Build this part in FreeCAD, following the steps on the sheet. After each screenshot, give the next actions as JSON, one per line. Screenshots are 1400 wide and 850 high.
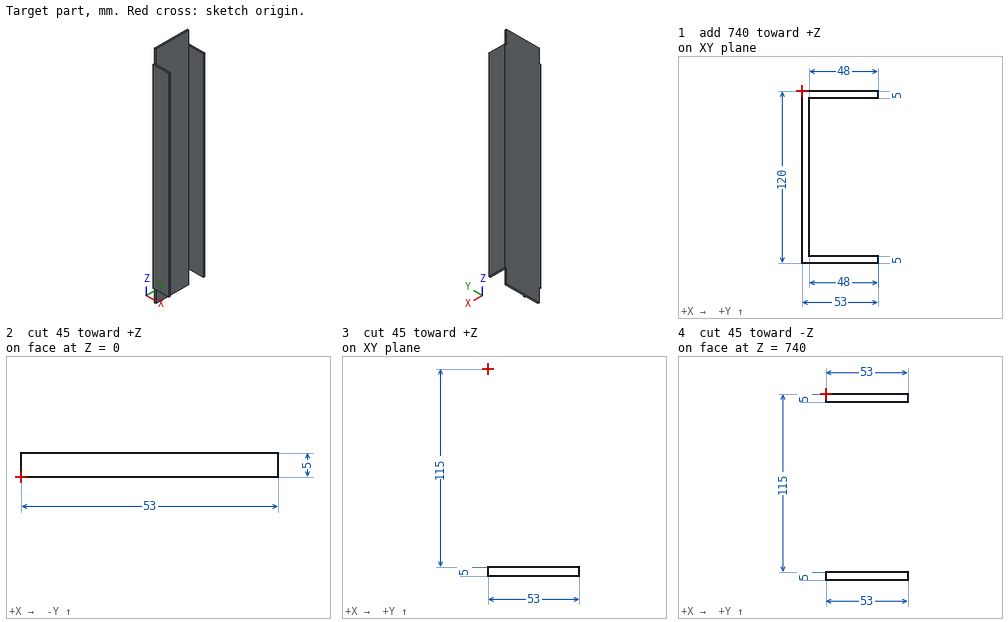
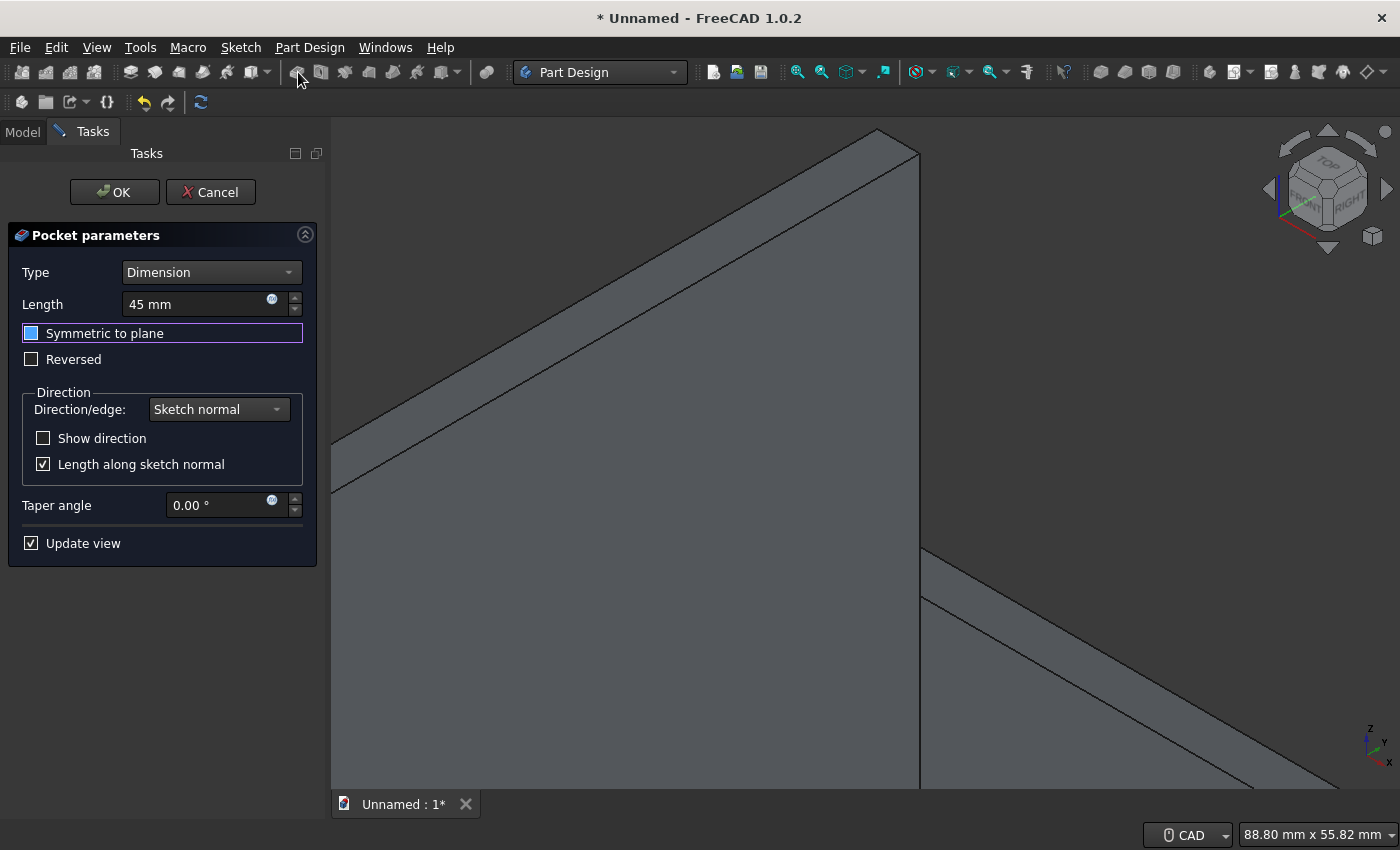
{"action": "left_click", "coordinate": [115, 192]}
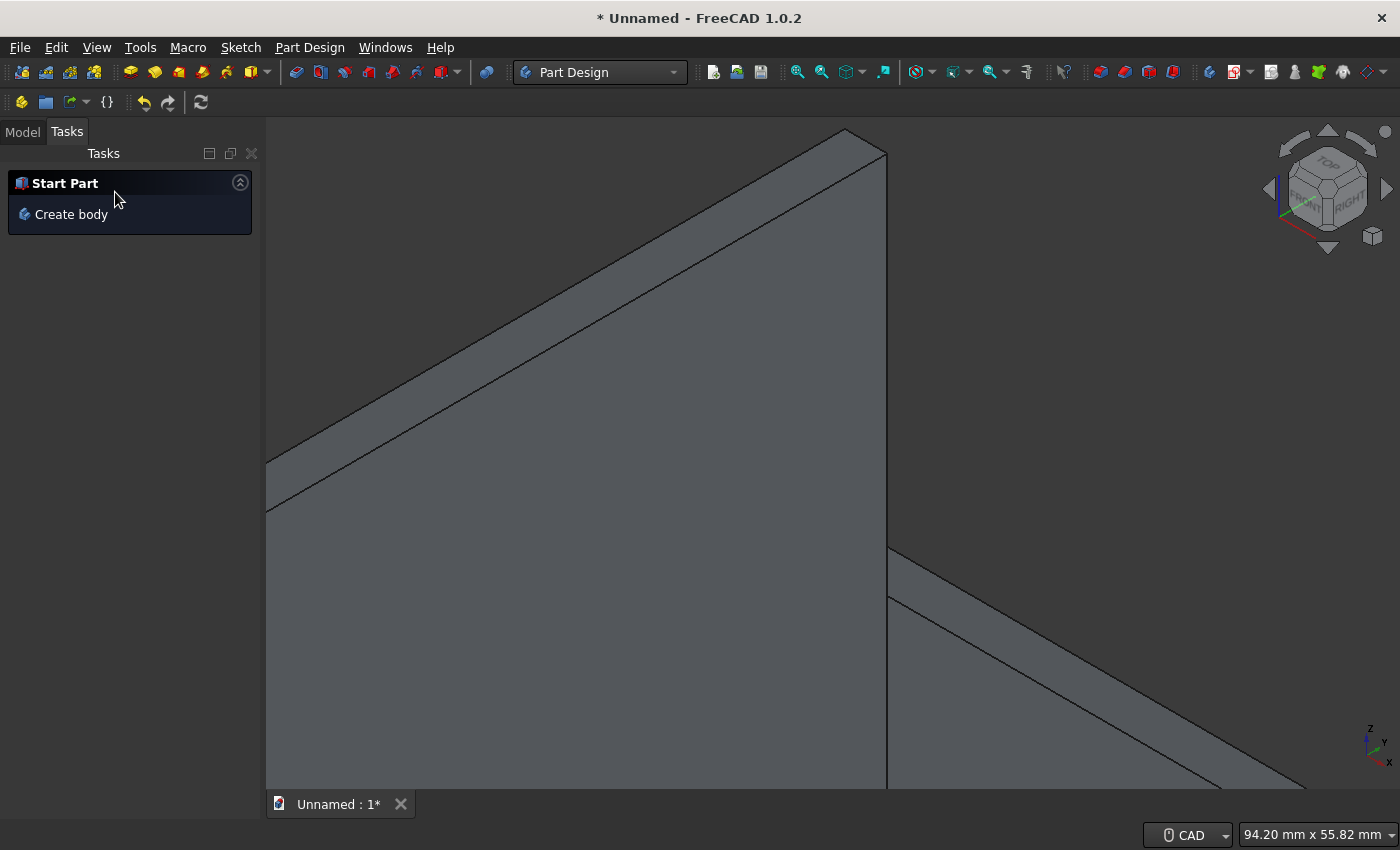
{"action": "left_click", "coordinate": [798, 72]}